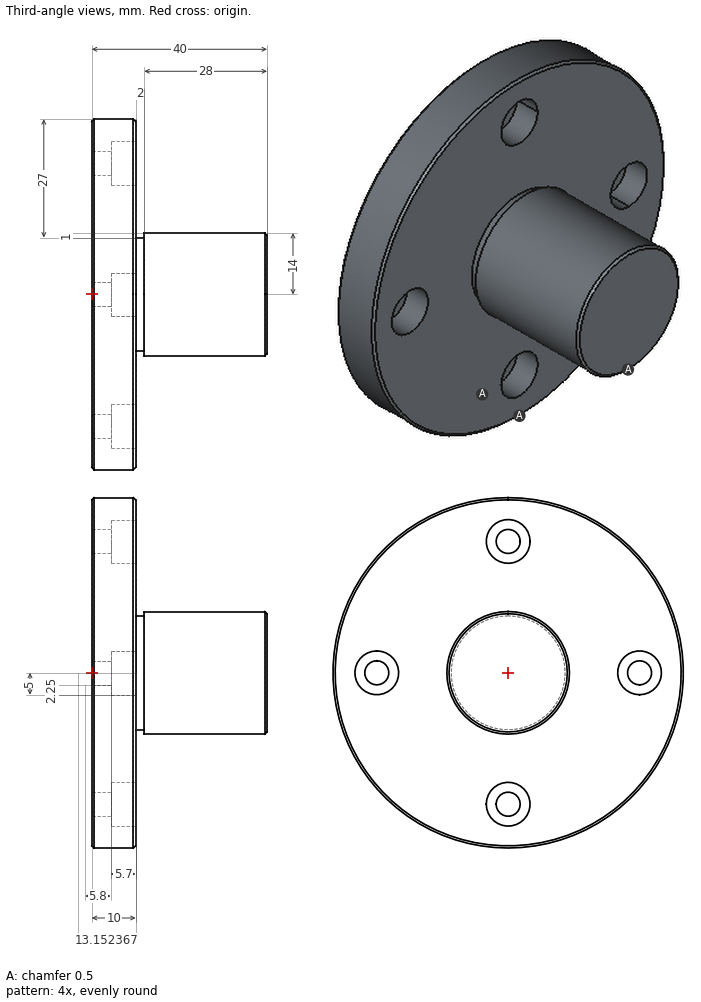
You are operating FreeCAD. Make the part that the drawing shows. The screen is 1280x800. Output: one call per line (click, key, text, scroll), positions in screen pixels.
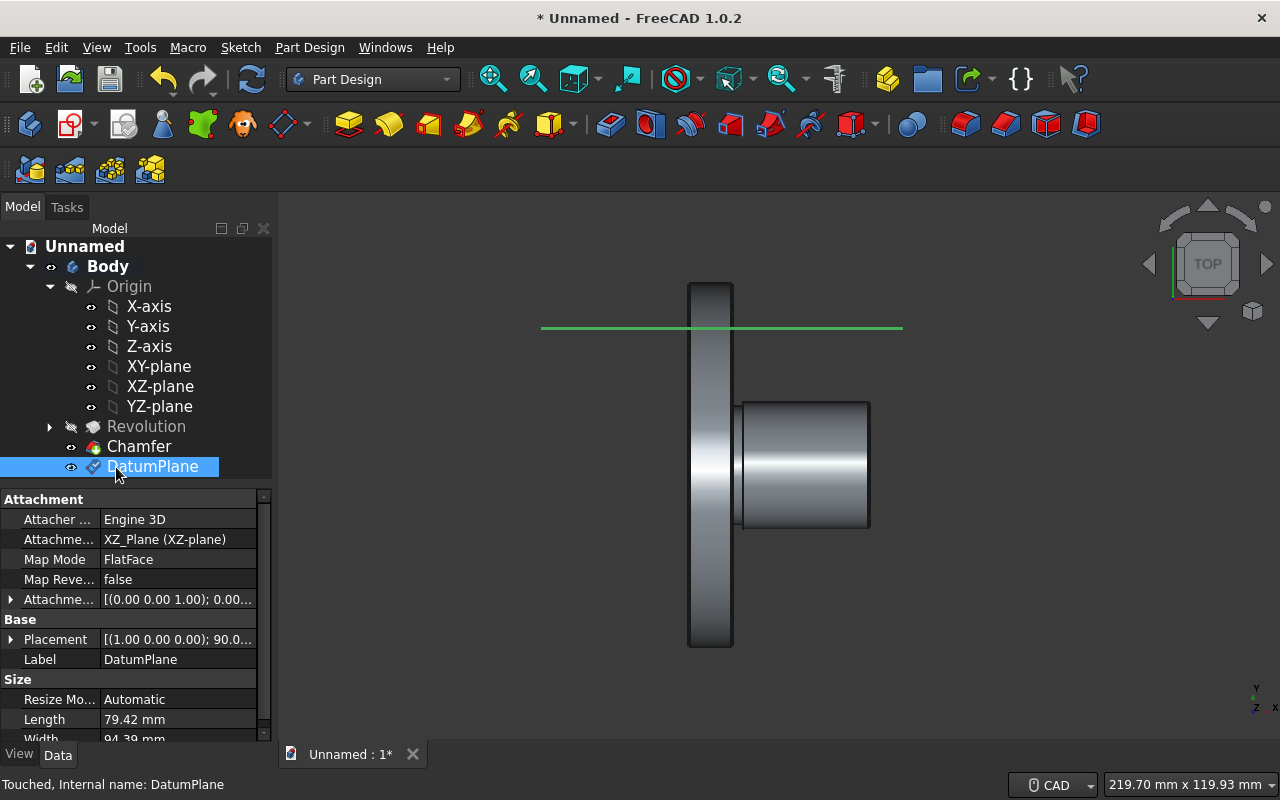
click(70, 124)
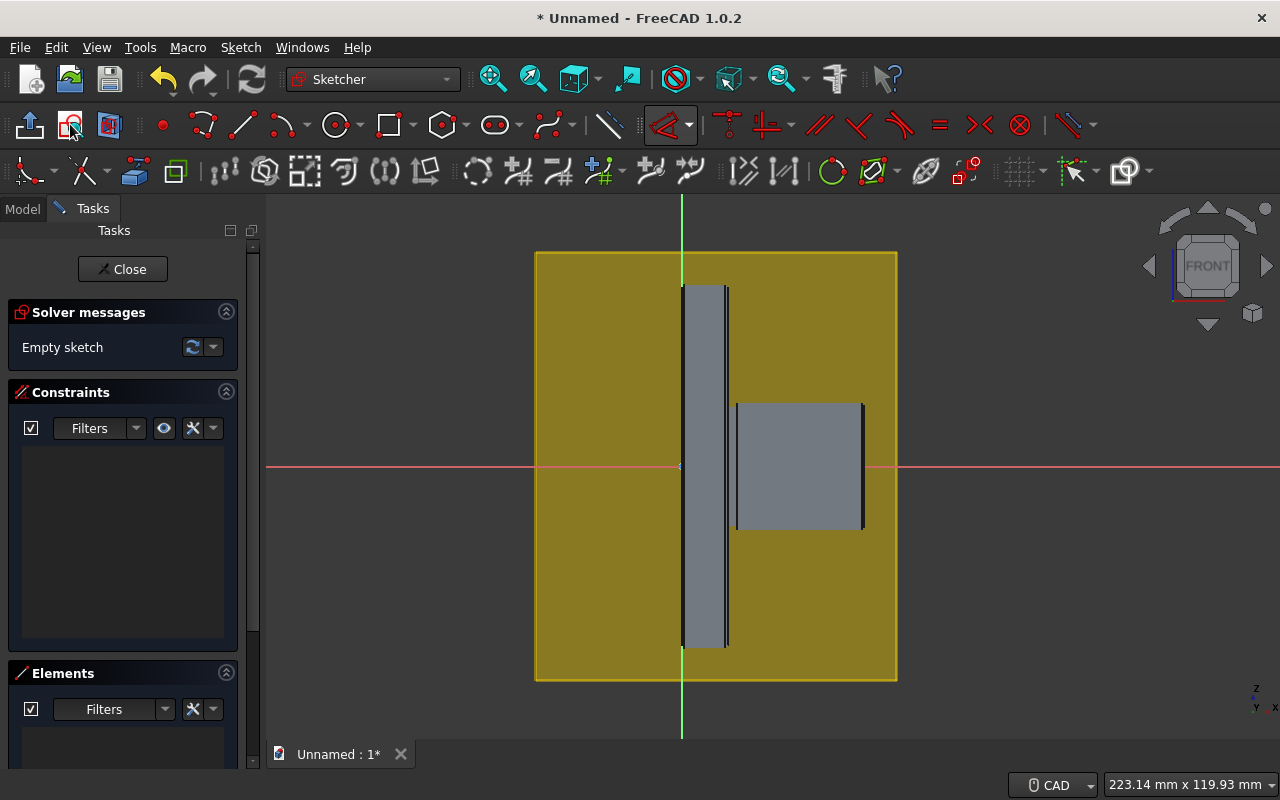
click(110, 126)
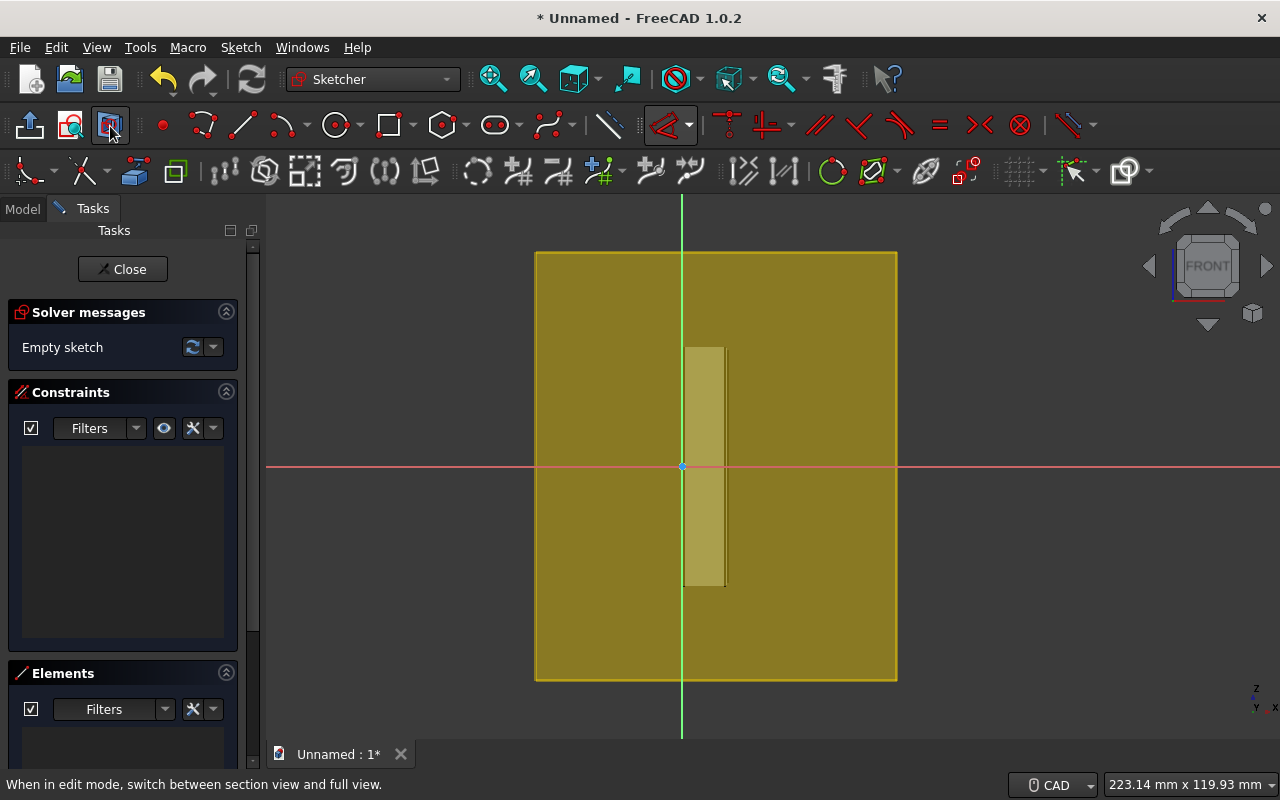
scroll(697, 479, up, 11)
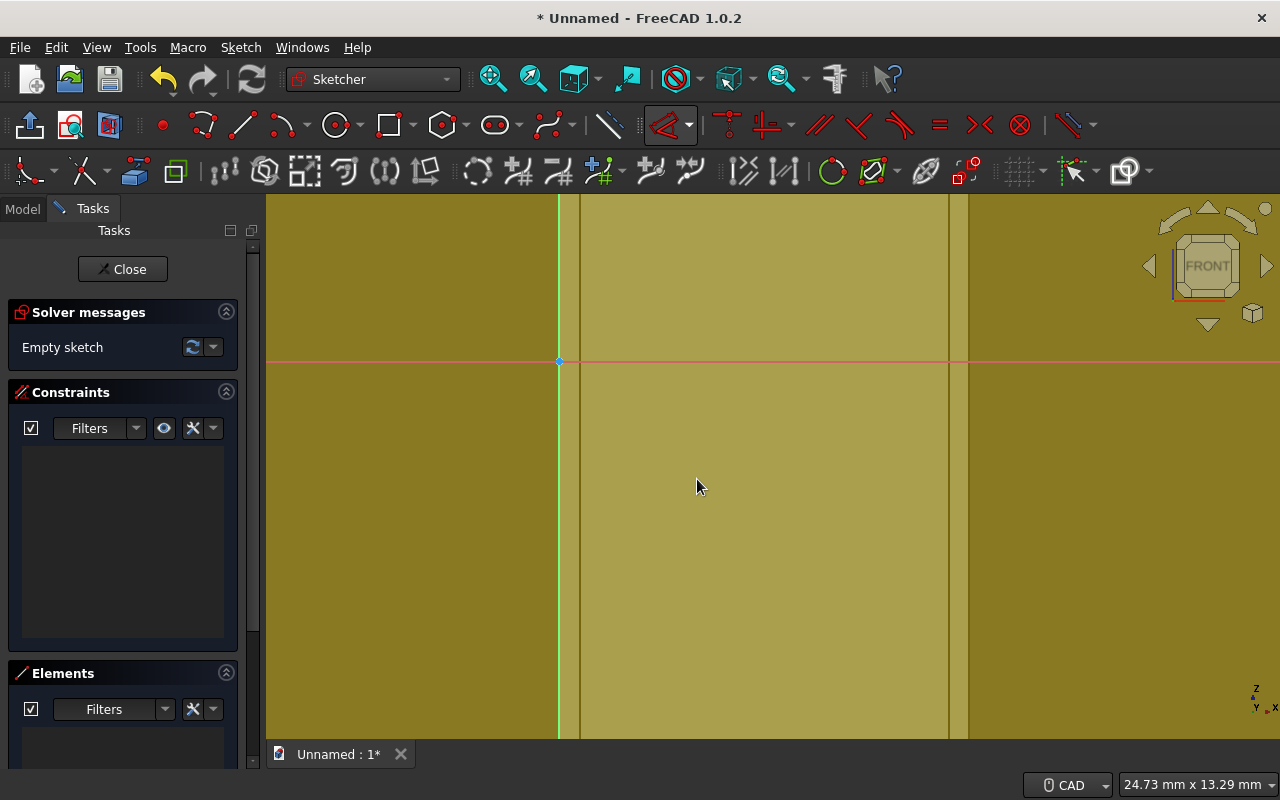
click(204, 126)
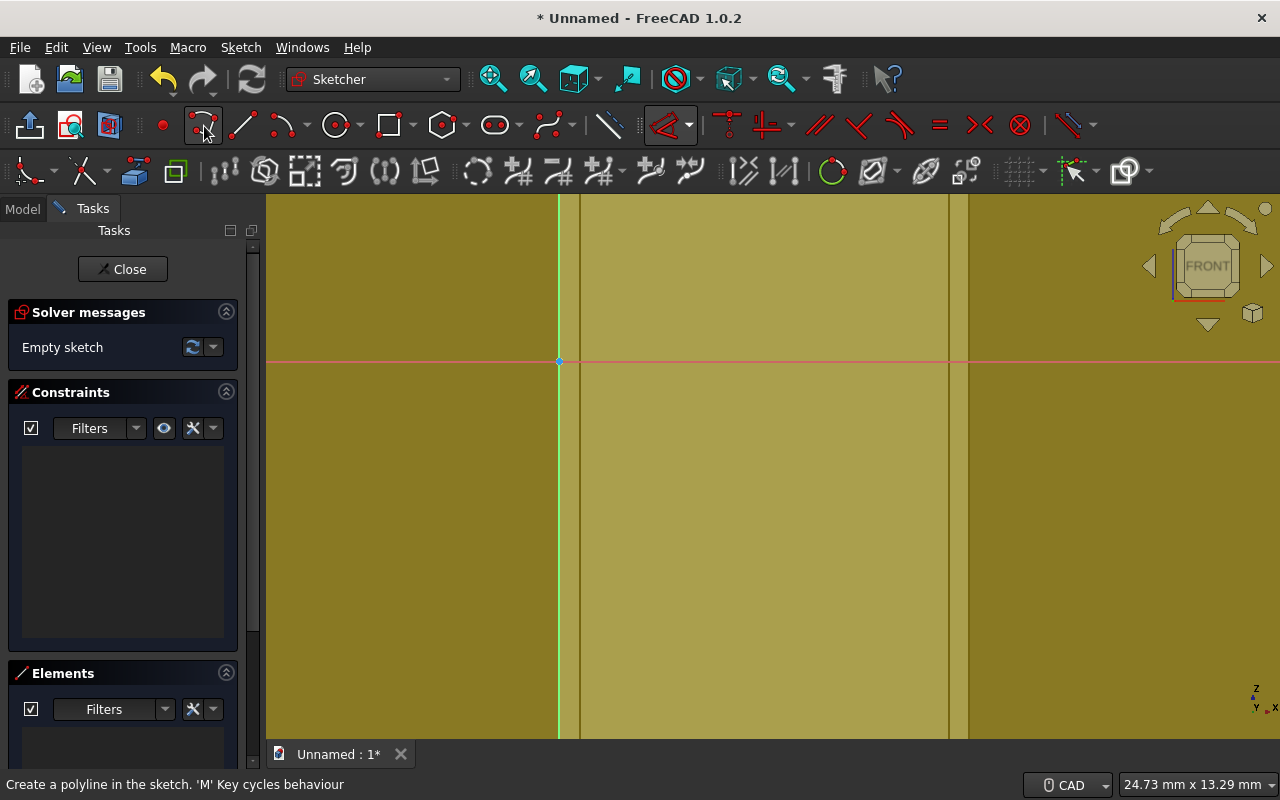
click(498, 475)
click(430, 362)
click(969, 371)
click(969, 567)
click(736, 567)
click(736, 475)
click(498, 476)
key(Escape)
key(Escape)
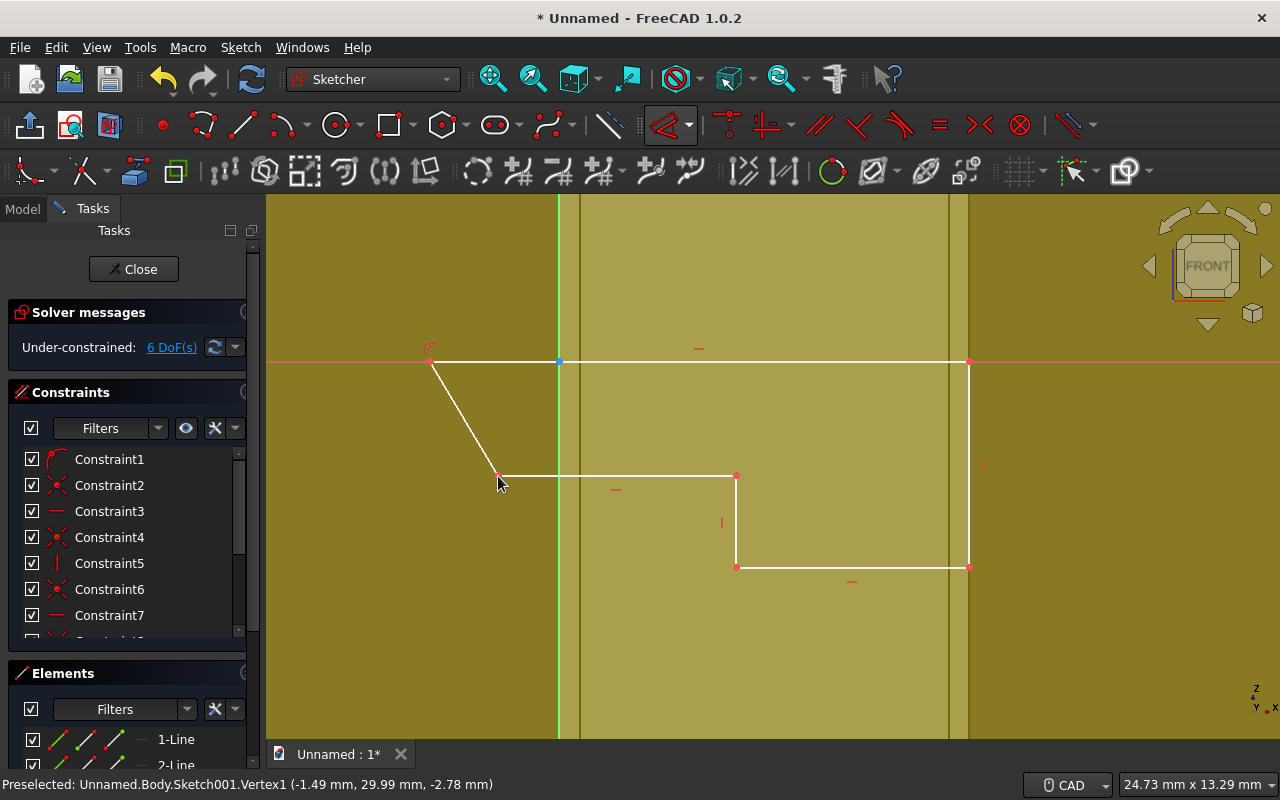
click(969, 424)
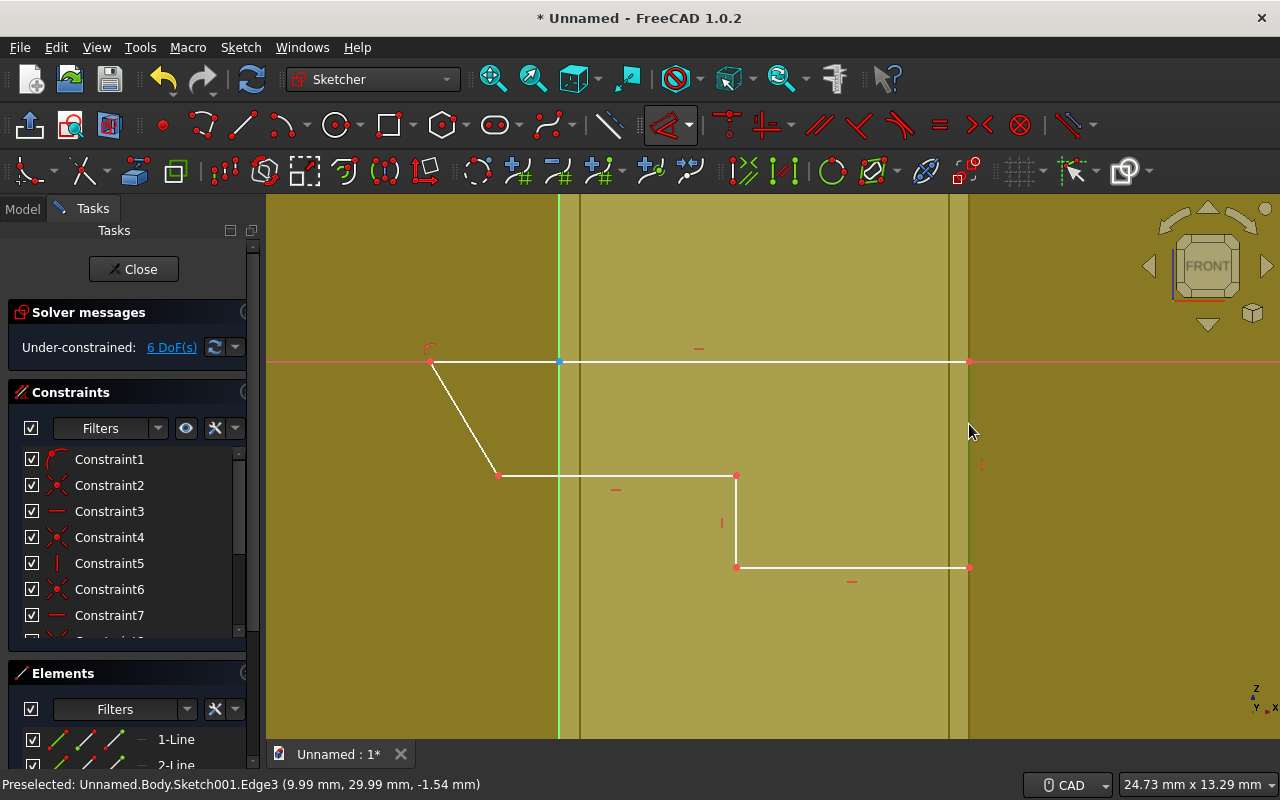
key(i)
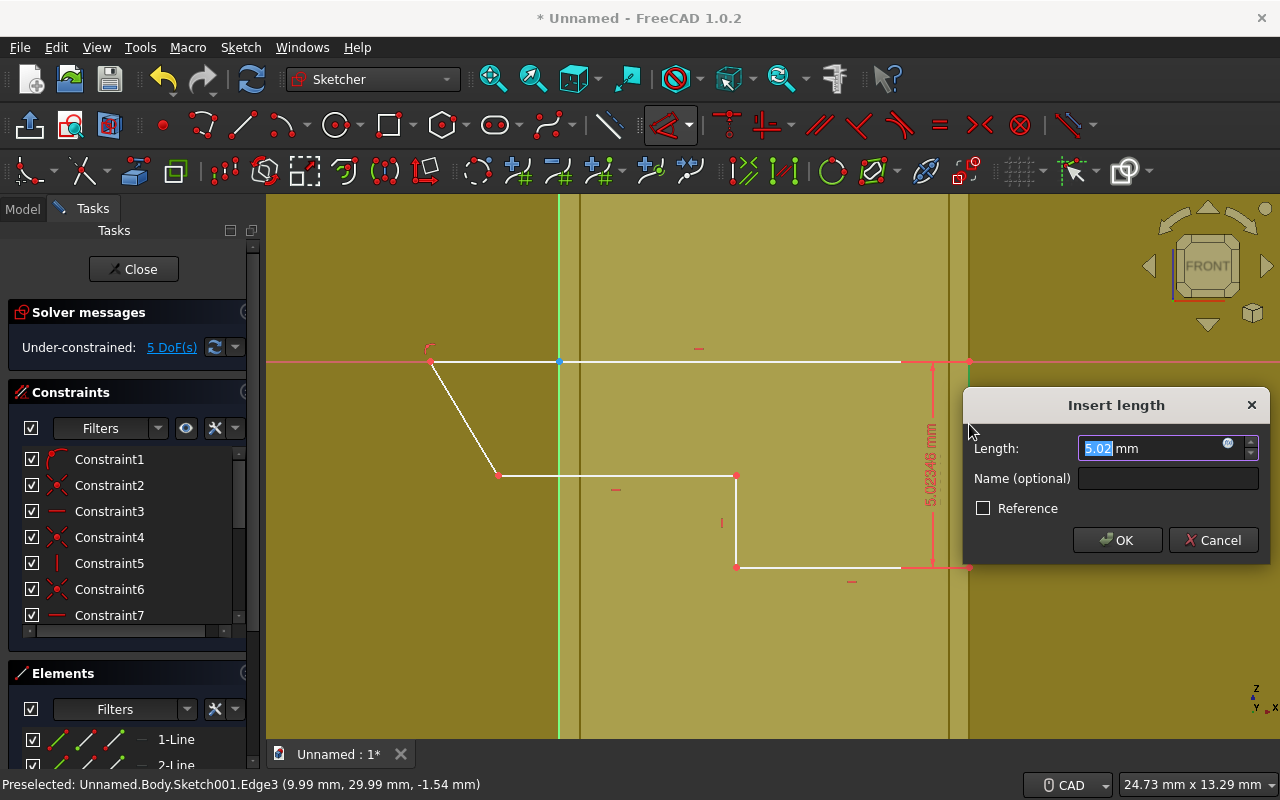
text(5)
key(Return)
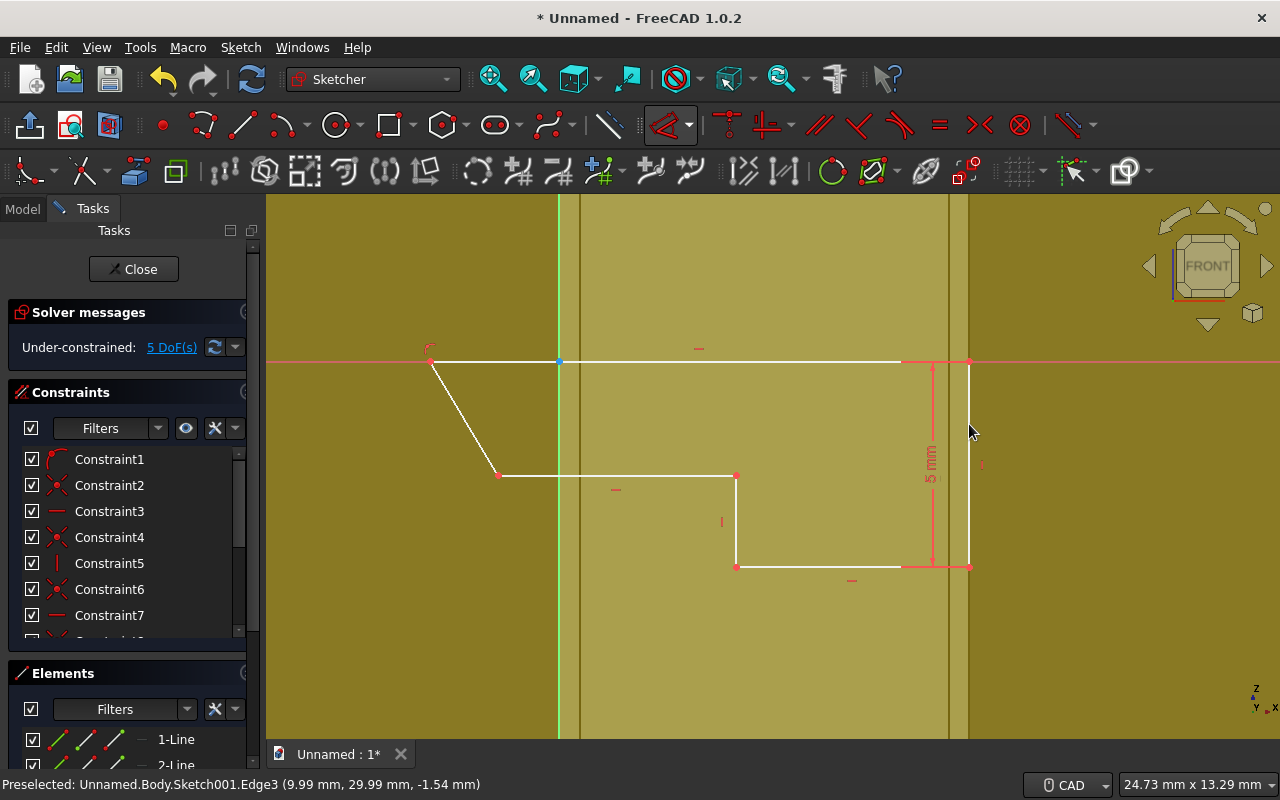
click(899, 567)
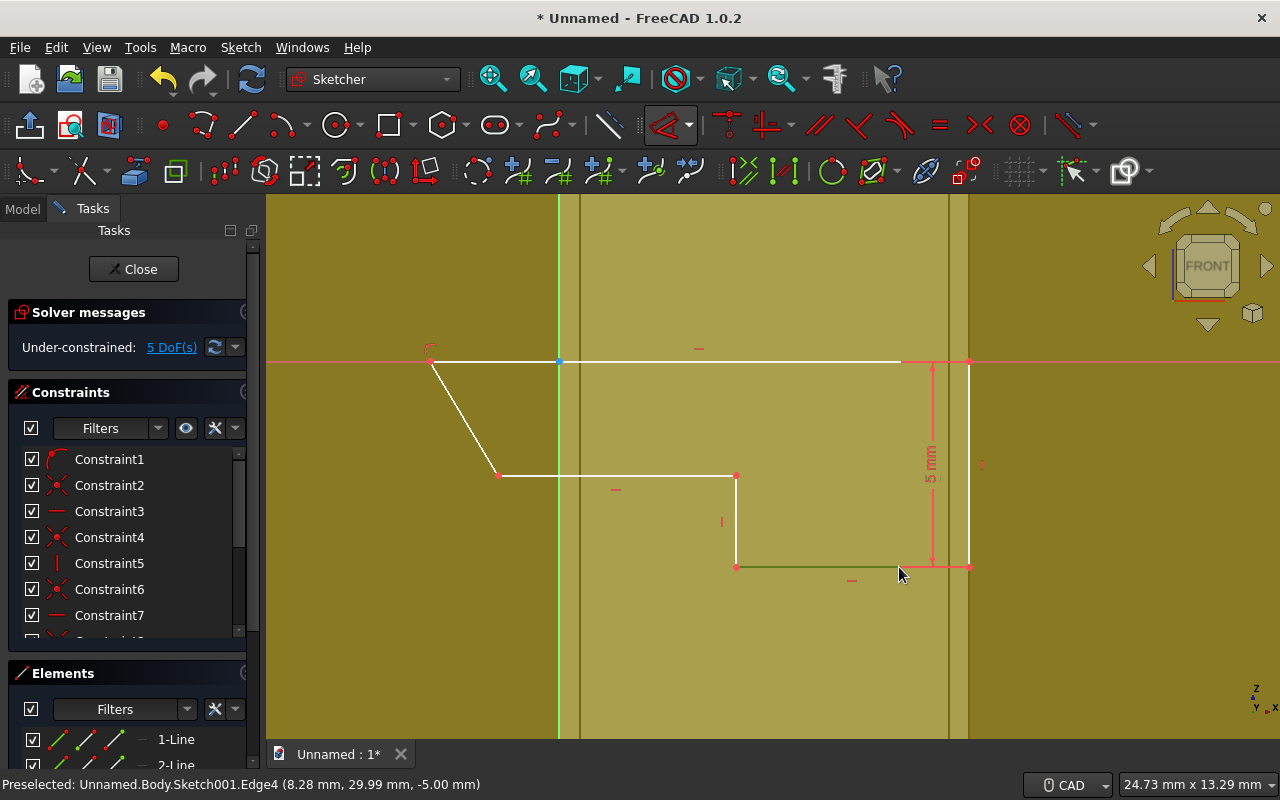
key(l)